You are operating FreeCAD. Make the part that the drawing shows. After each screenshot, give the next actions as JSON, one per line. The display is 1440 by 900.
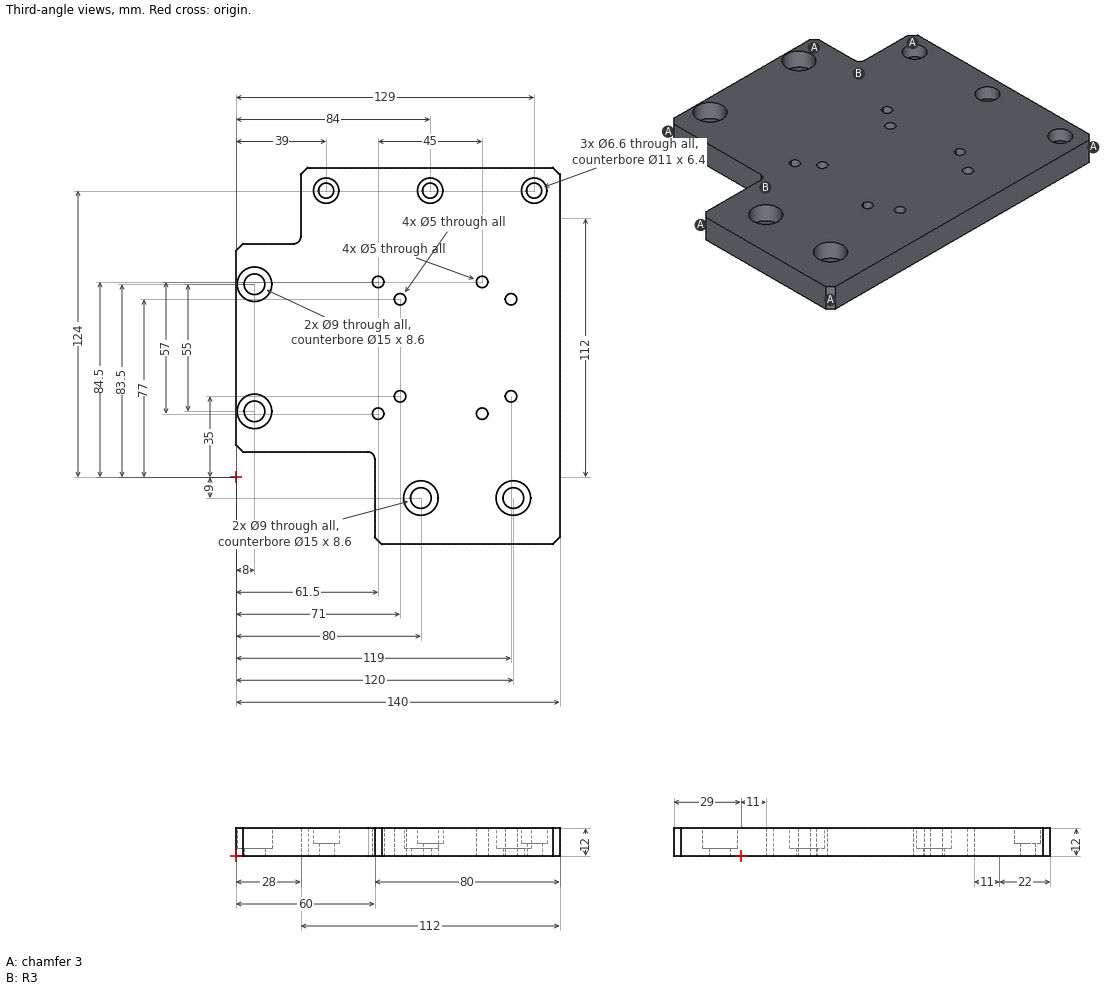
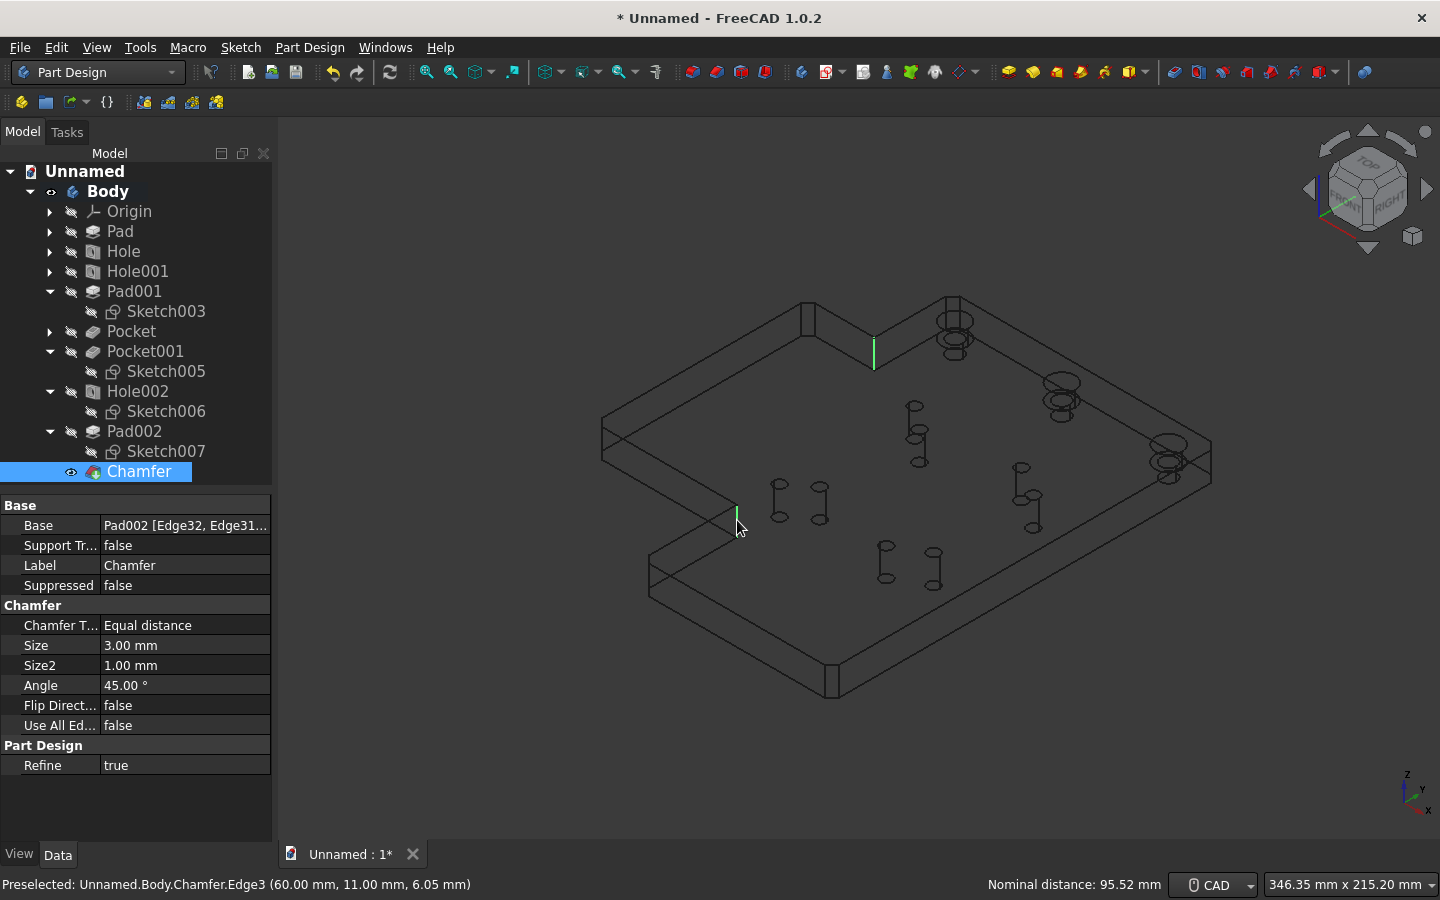
{"action": "key", "text": "v 1"}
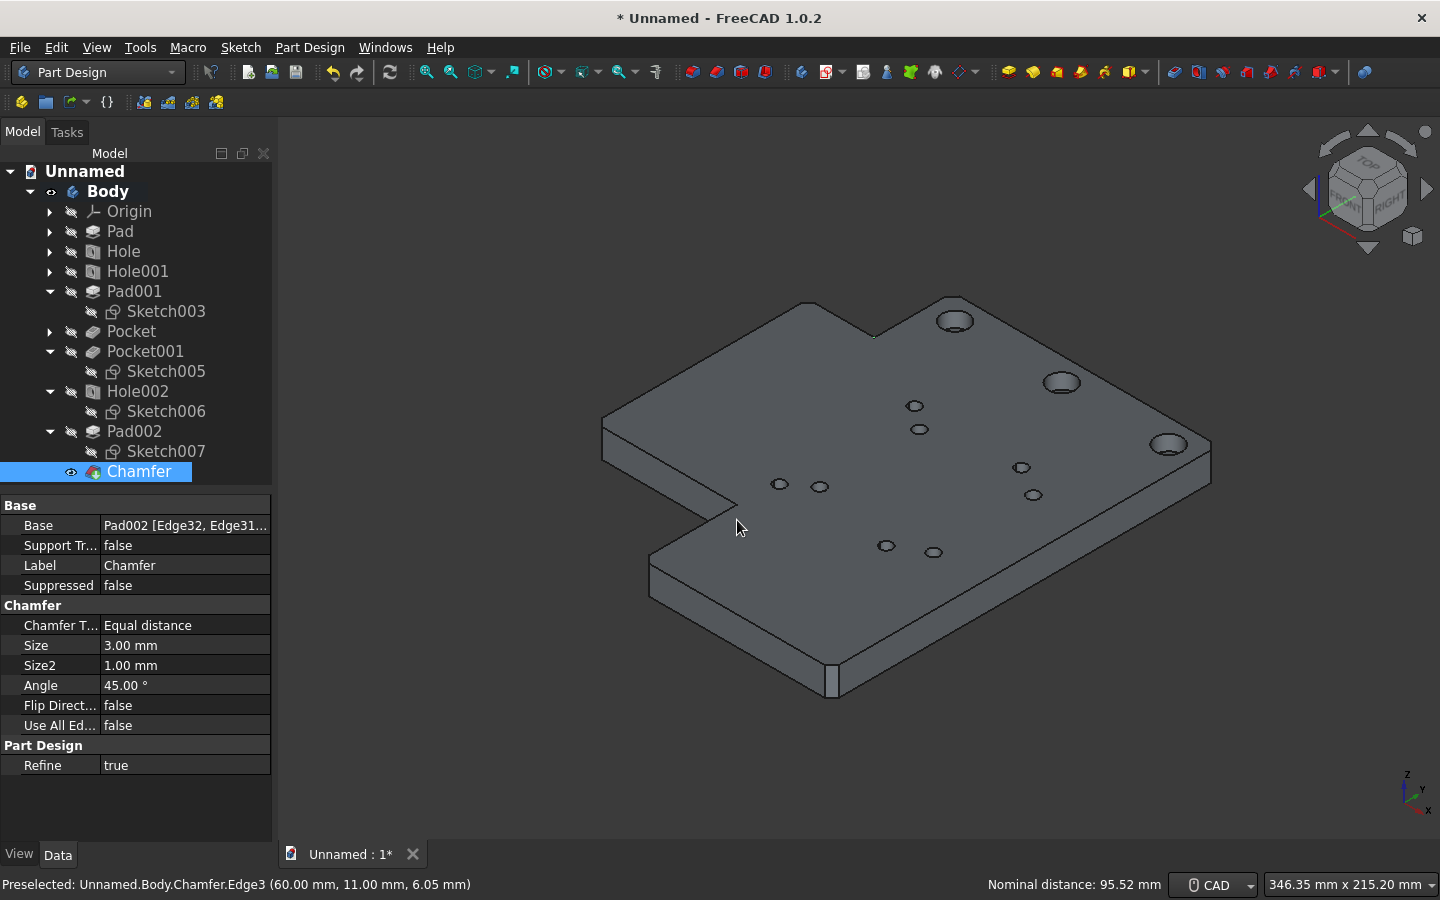
{"action": "left_click", "coordinate": [694, 72]}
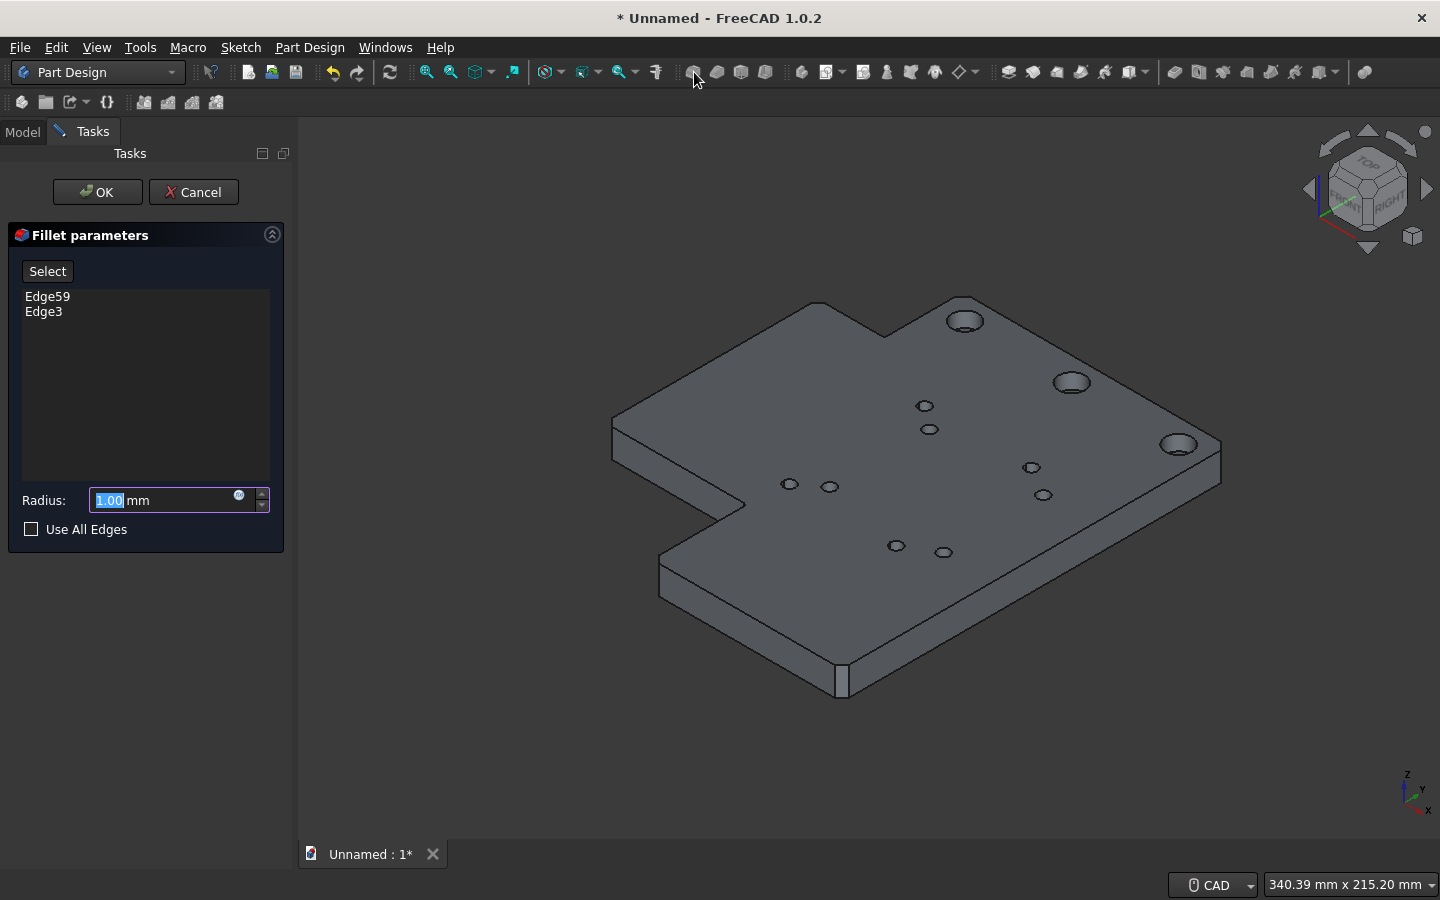
{"action": "type", "text": "3"}
{"action": "key", "text": "Tab"}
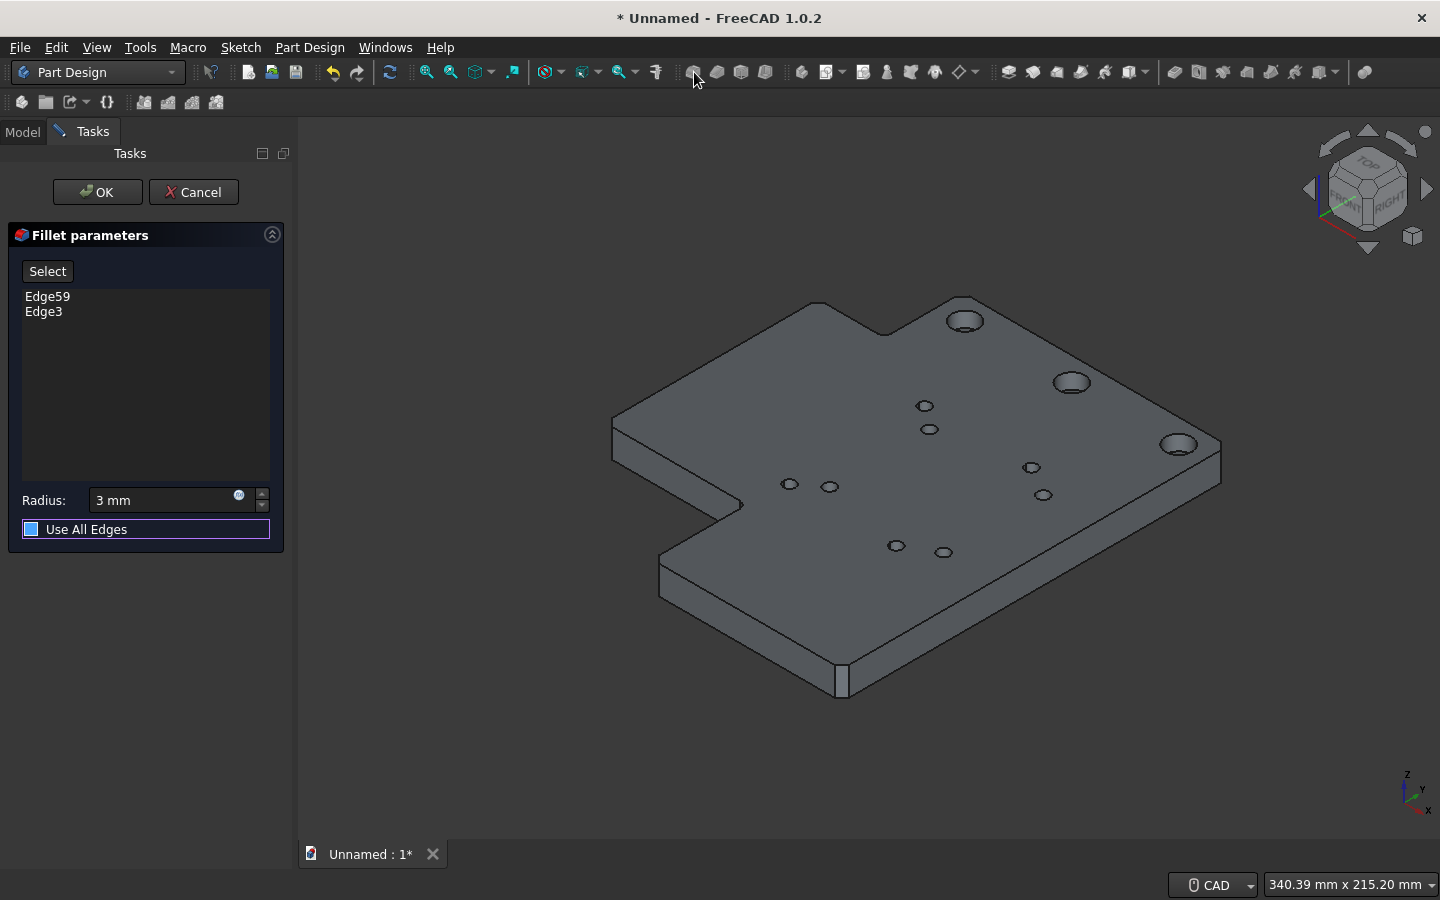
{"action": "left_click", "coordinate": [98, 192]}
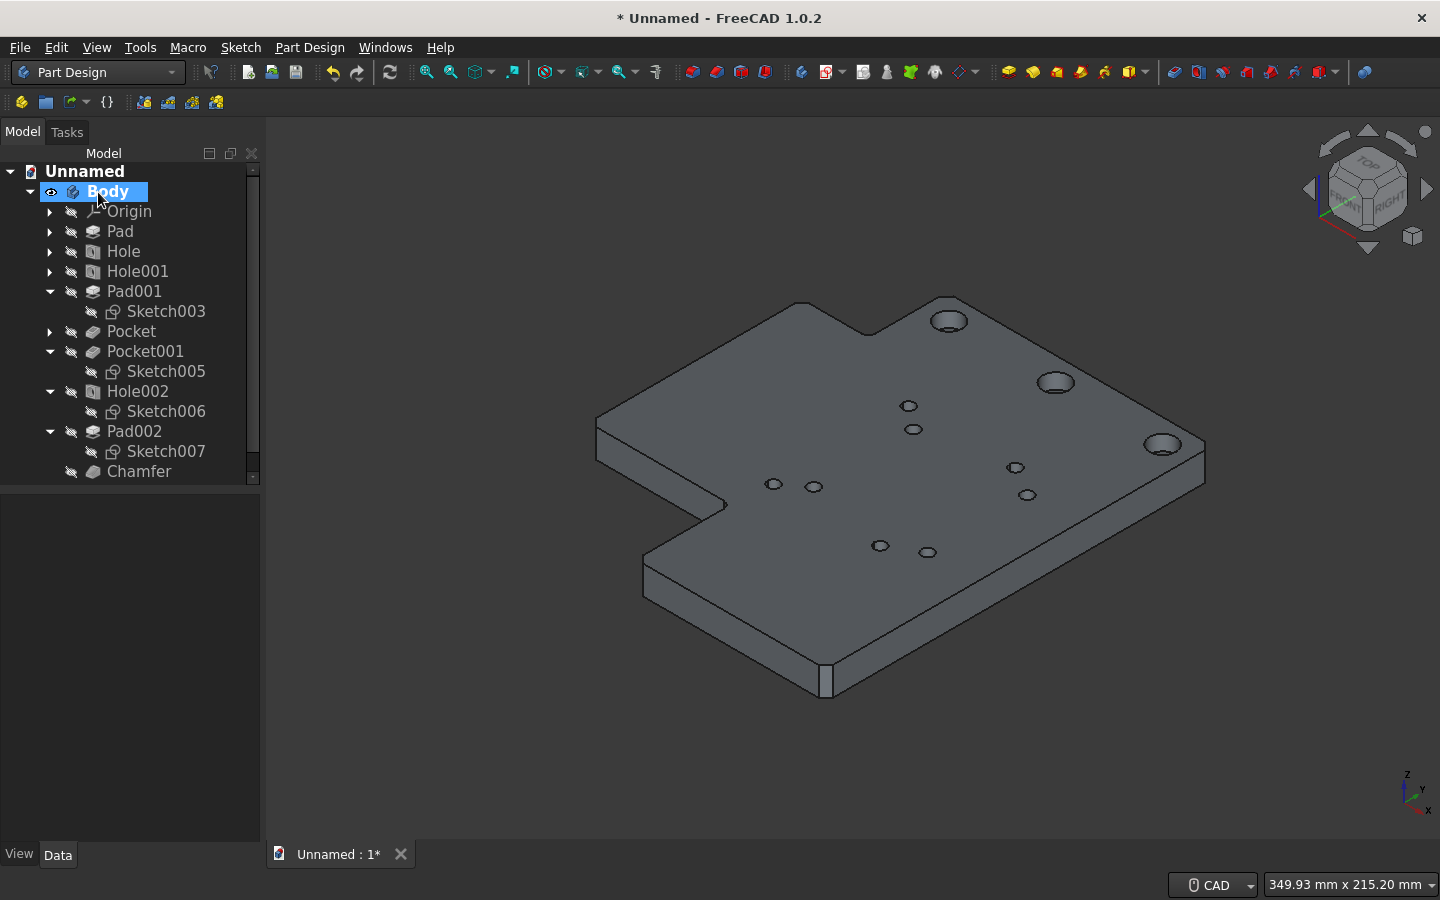
{"action": "left_click", "coordinate": [758, 406]}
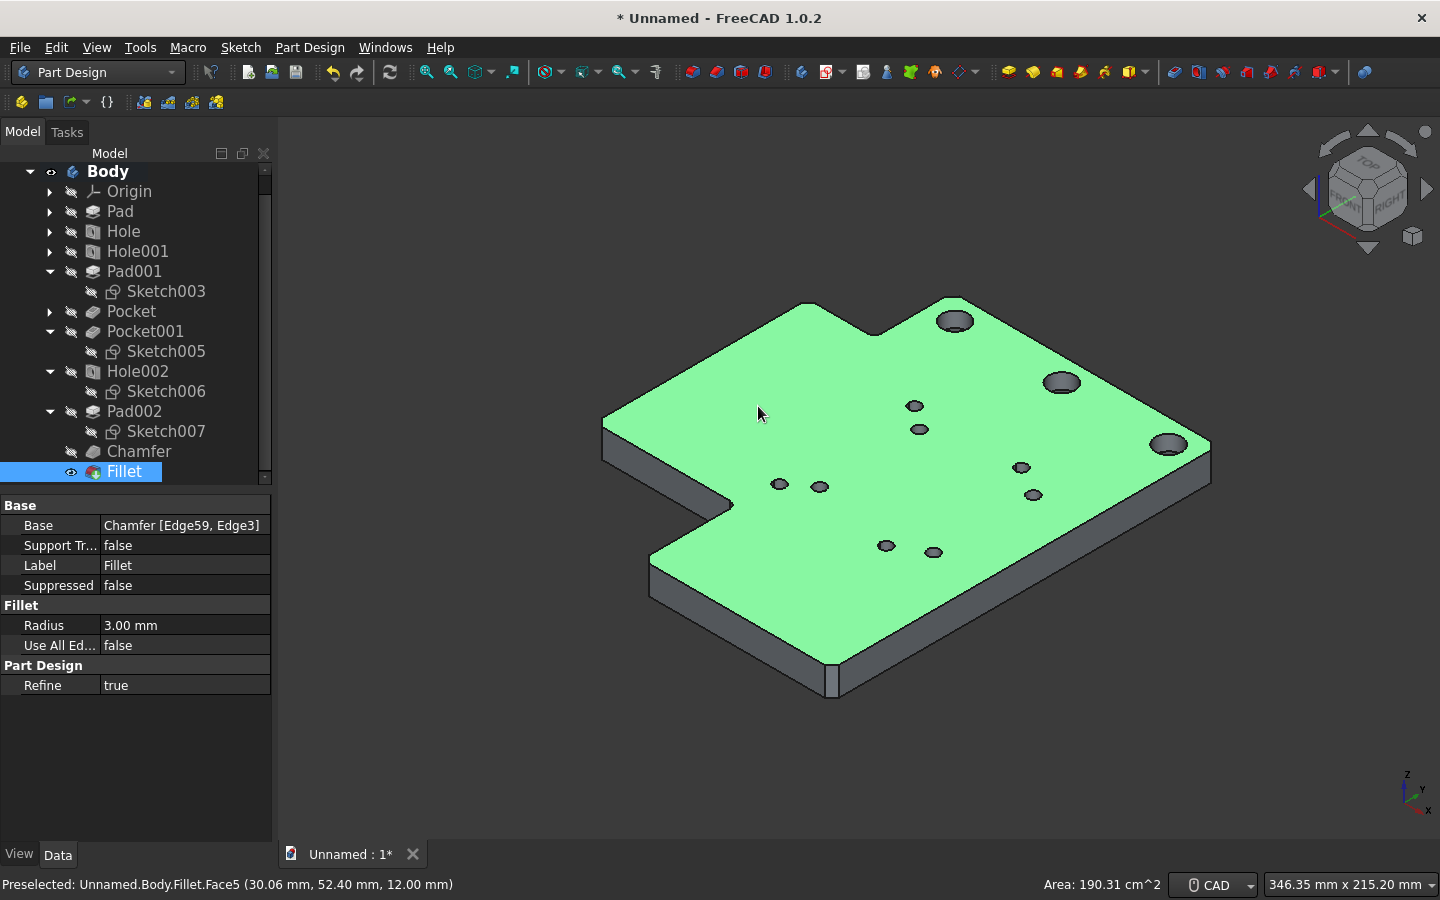
{"action": "left_click", "coordinate": [826, 72]}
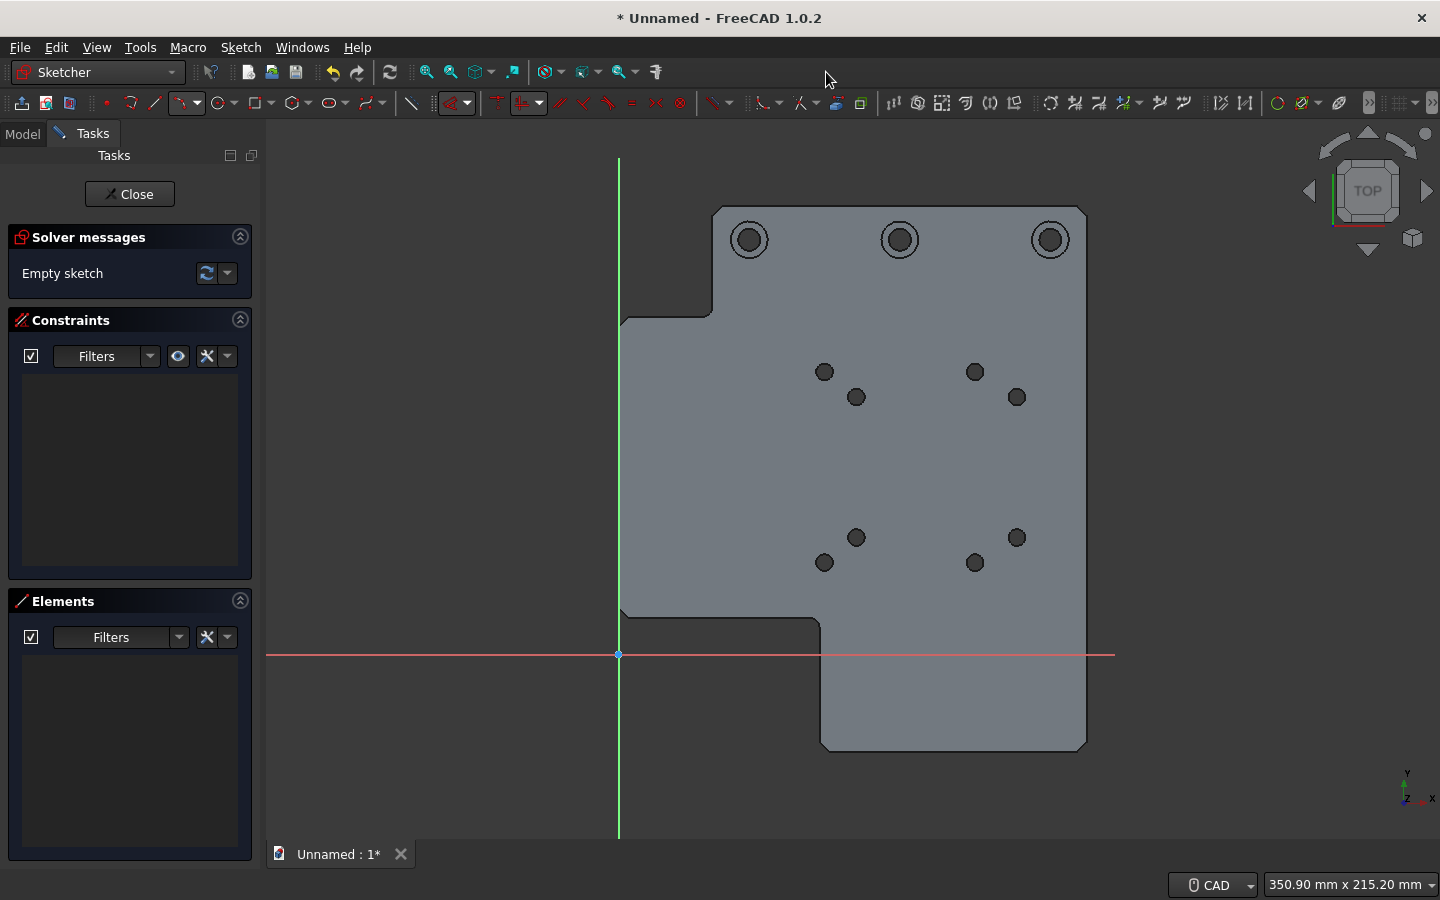
{"action": "scroll", "coordinate": [345, 565], "scroll_direction": "up", "scroll_amount": 2}